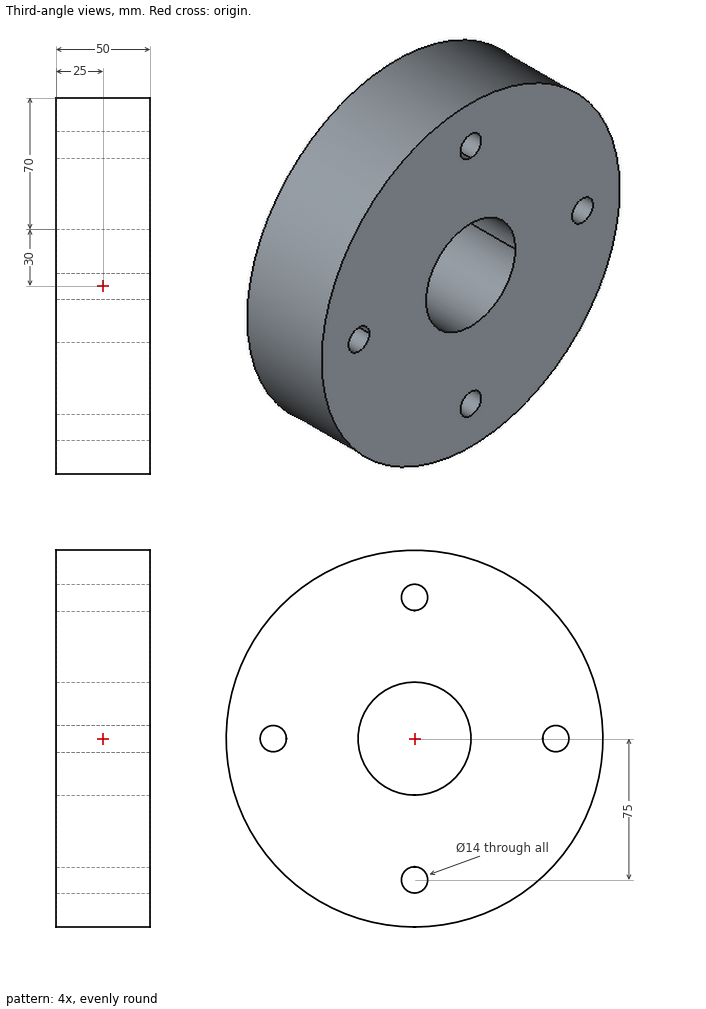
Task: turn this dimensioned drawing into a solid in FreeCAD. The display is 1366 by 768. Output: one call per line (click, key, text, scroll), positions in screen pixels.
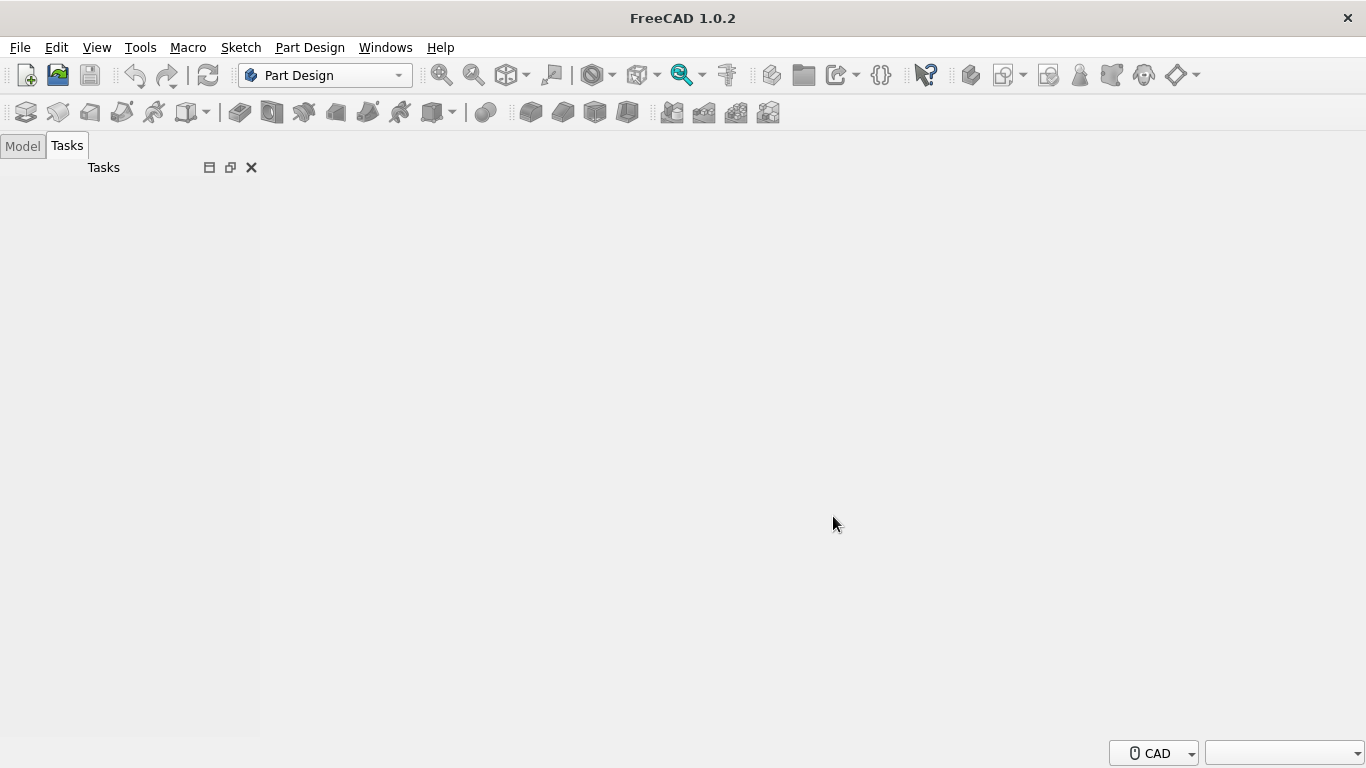
click(26, 76)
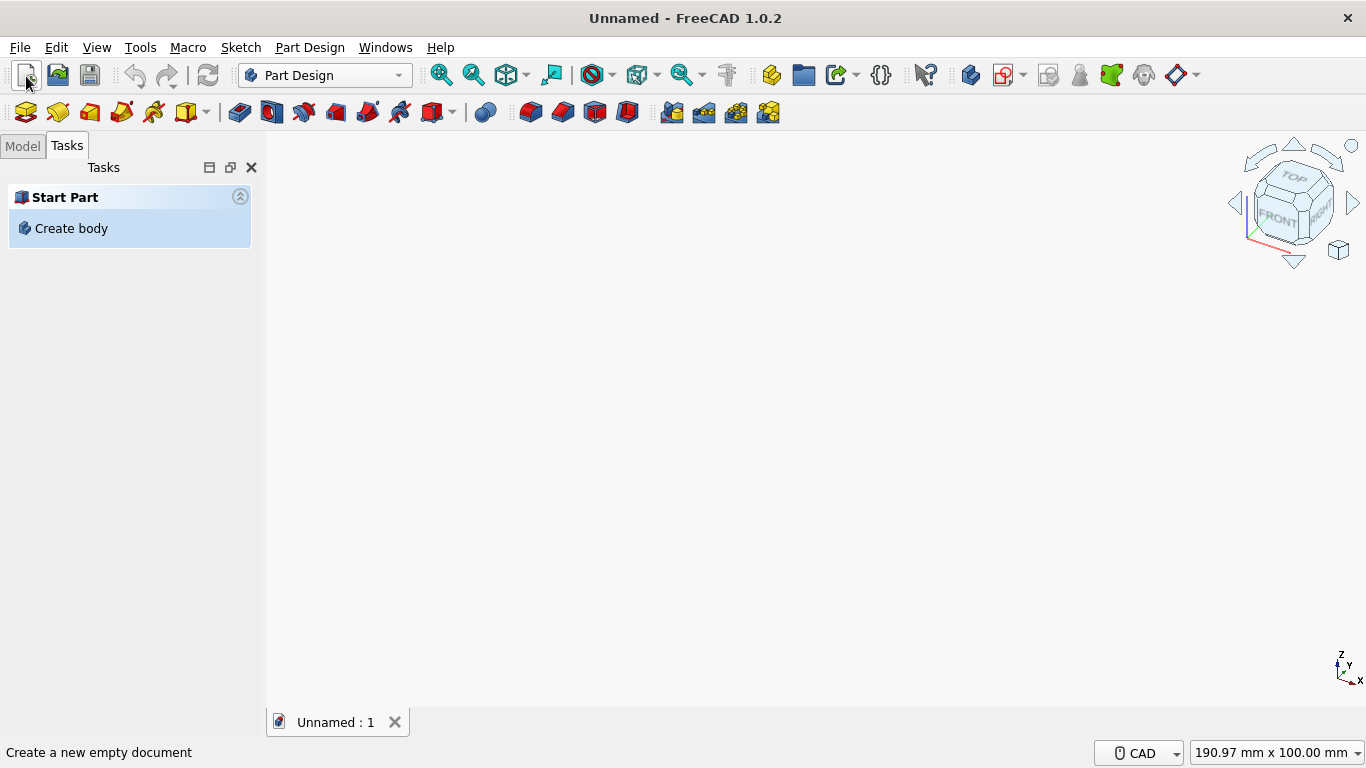
click(1004, 76)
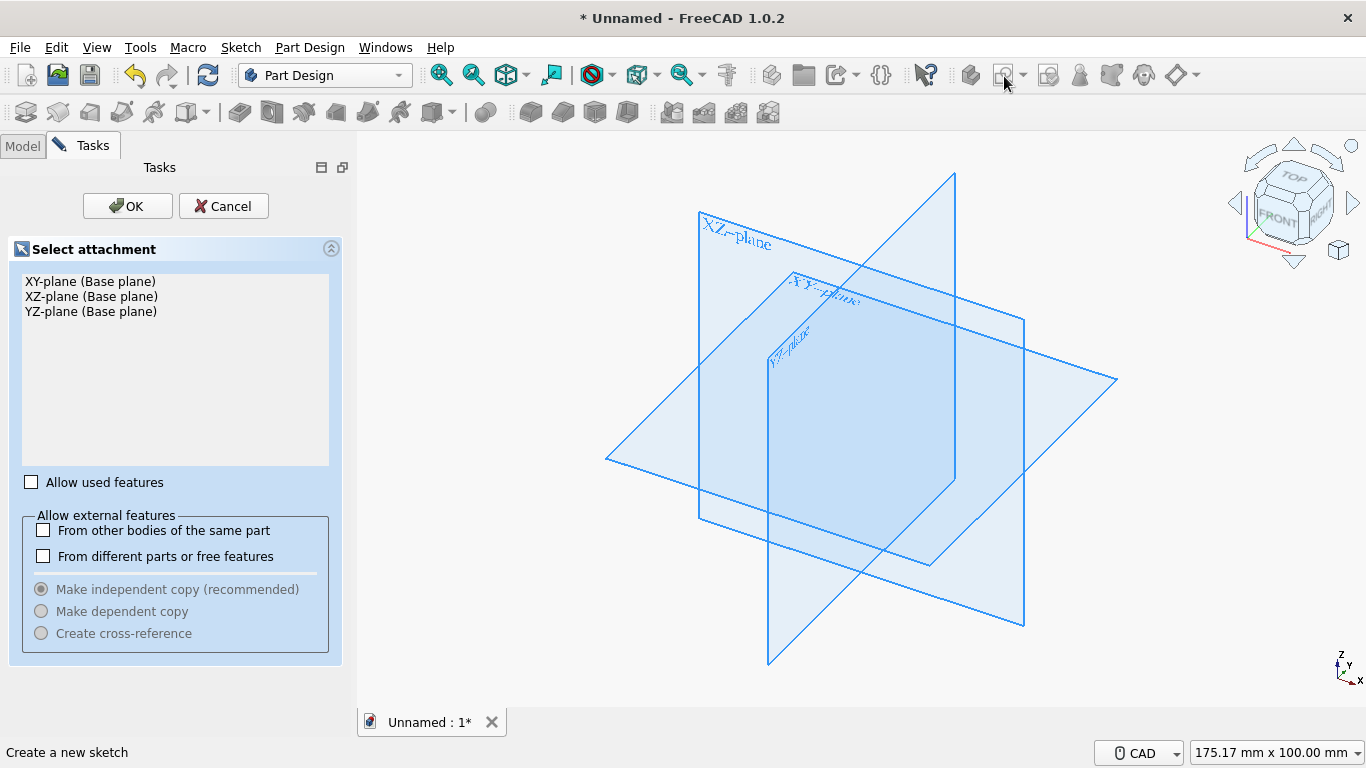
click(82, 282)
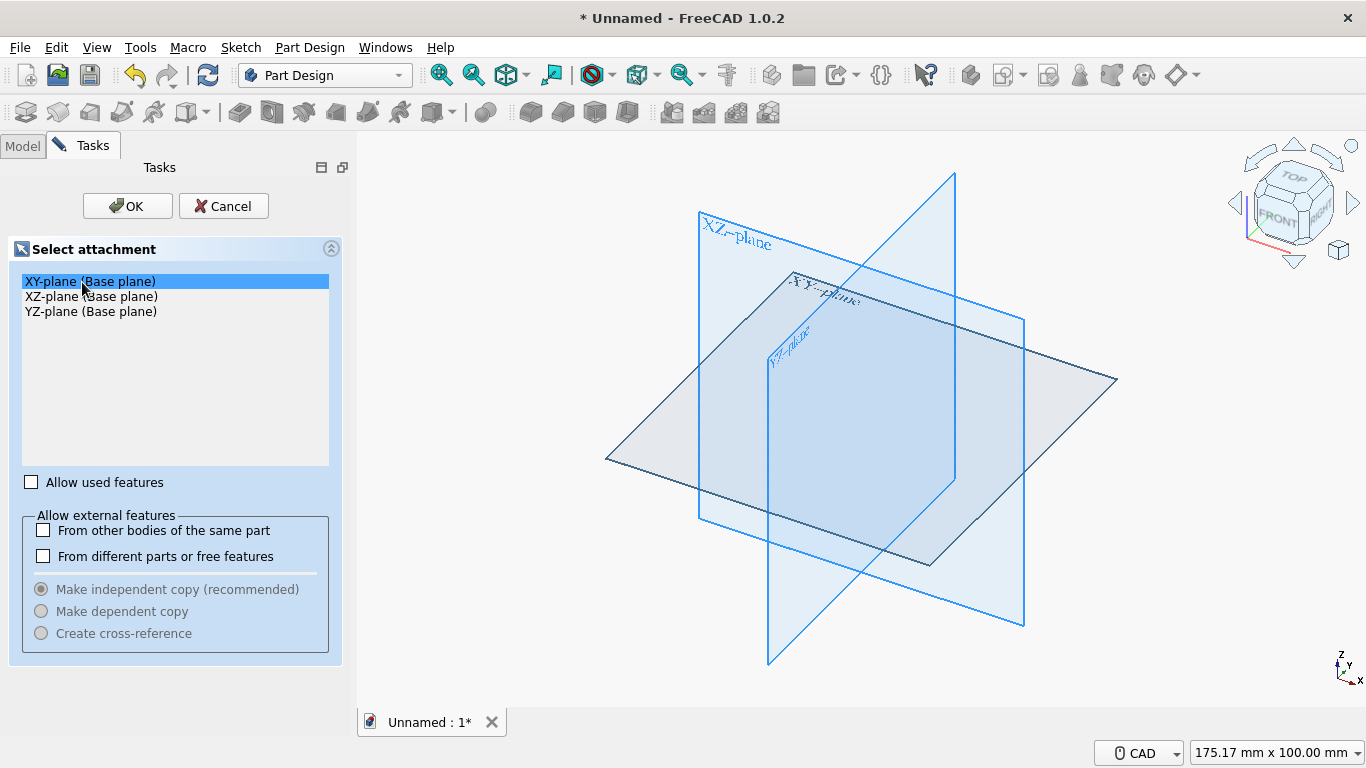
click(128, 206)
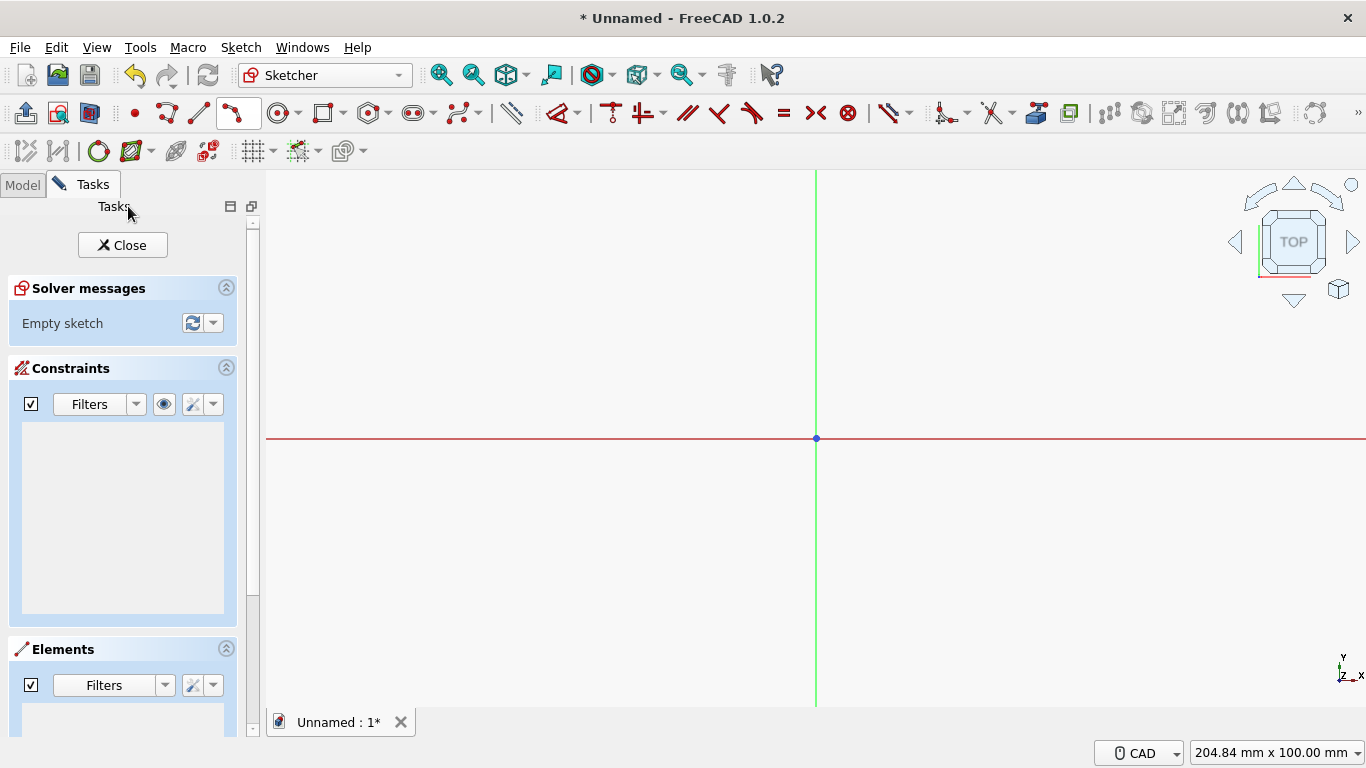
scroll(664, 679, down, 3)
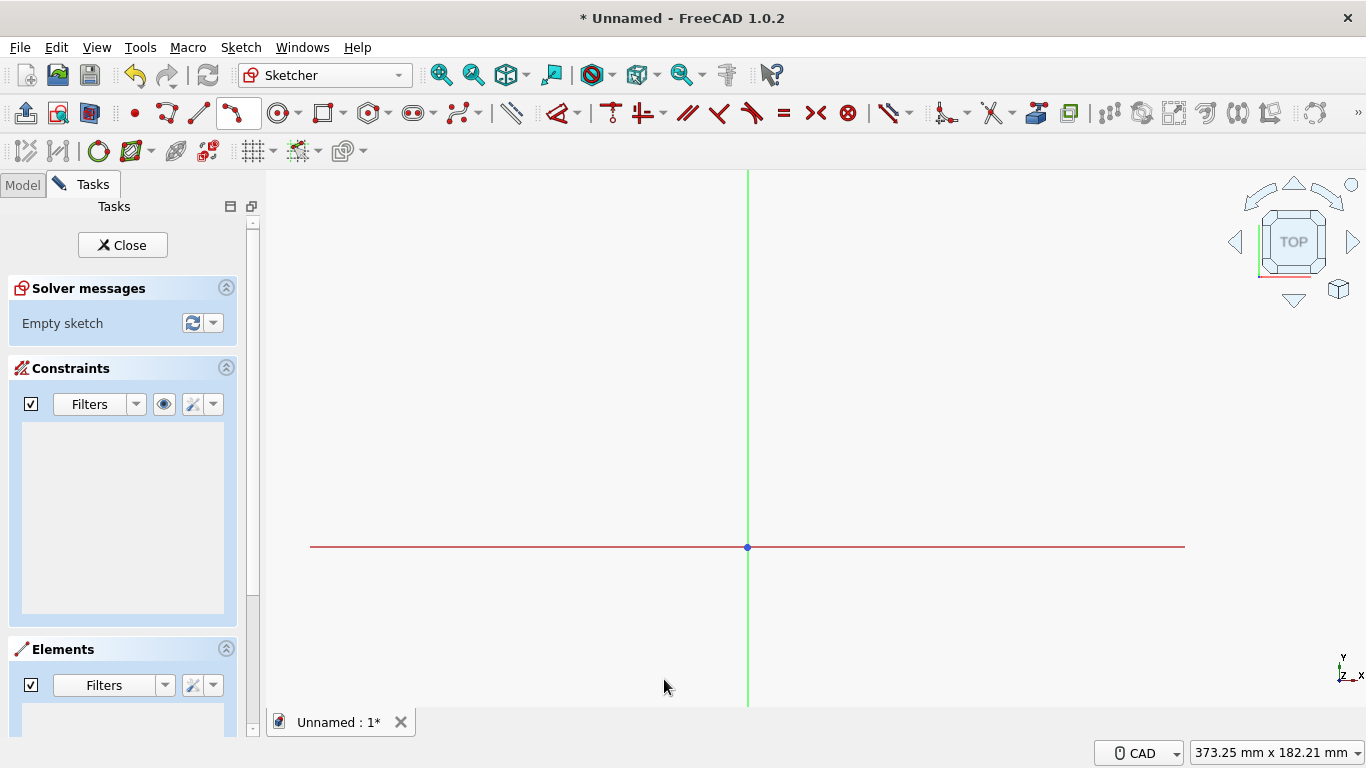
click(324, 114)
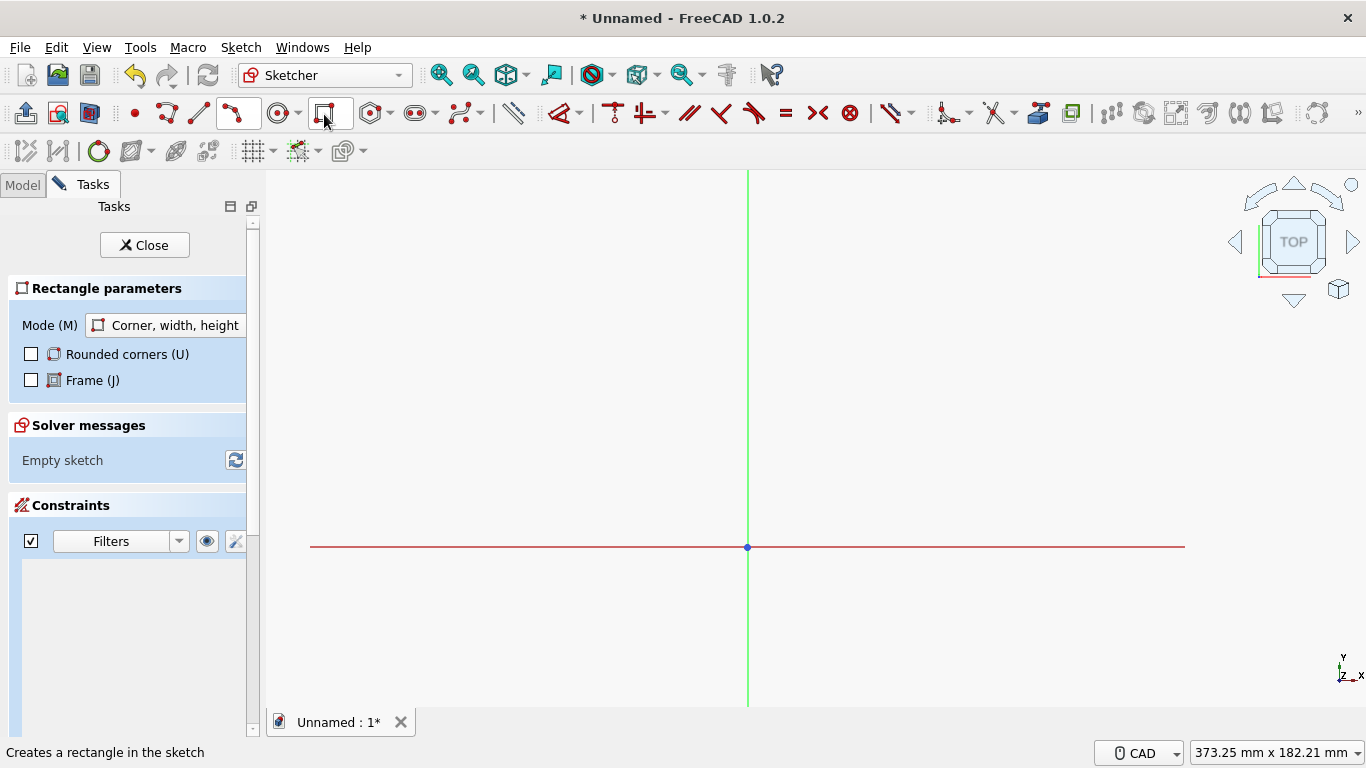
click(674, 253)
click(821, 459)
key(Escape)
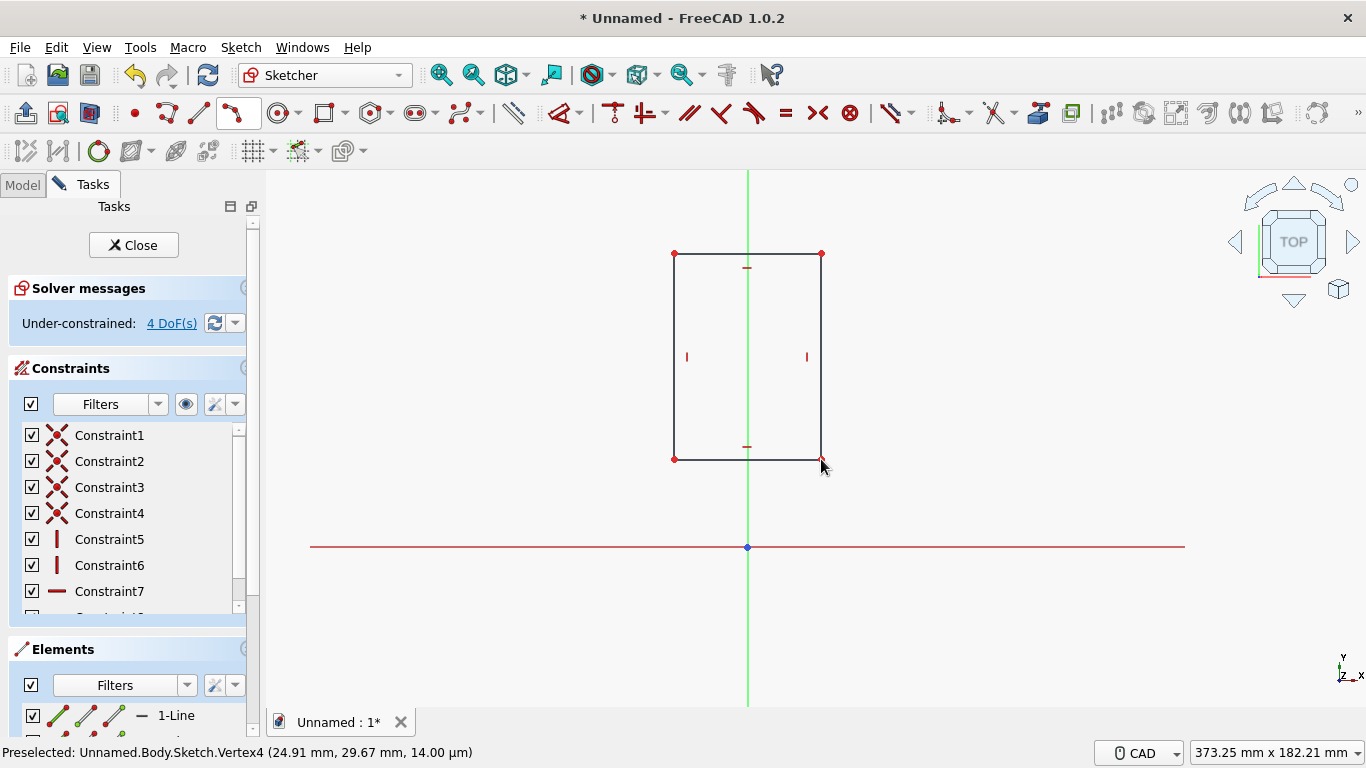
click(560, 114)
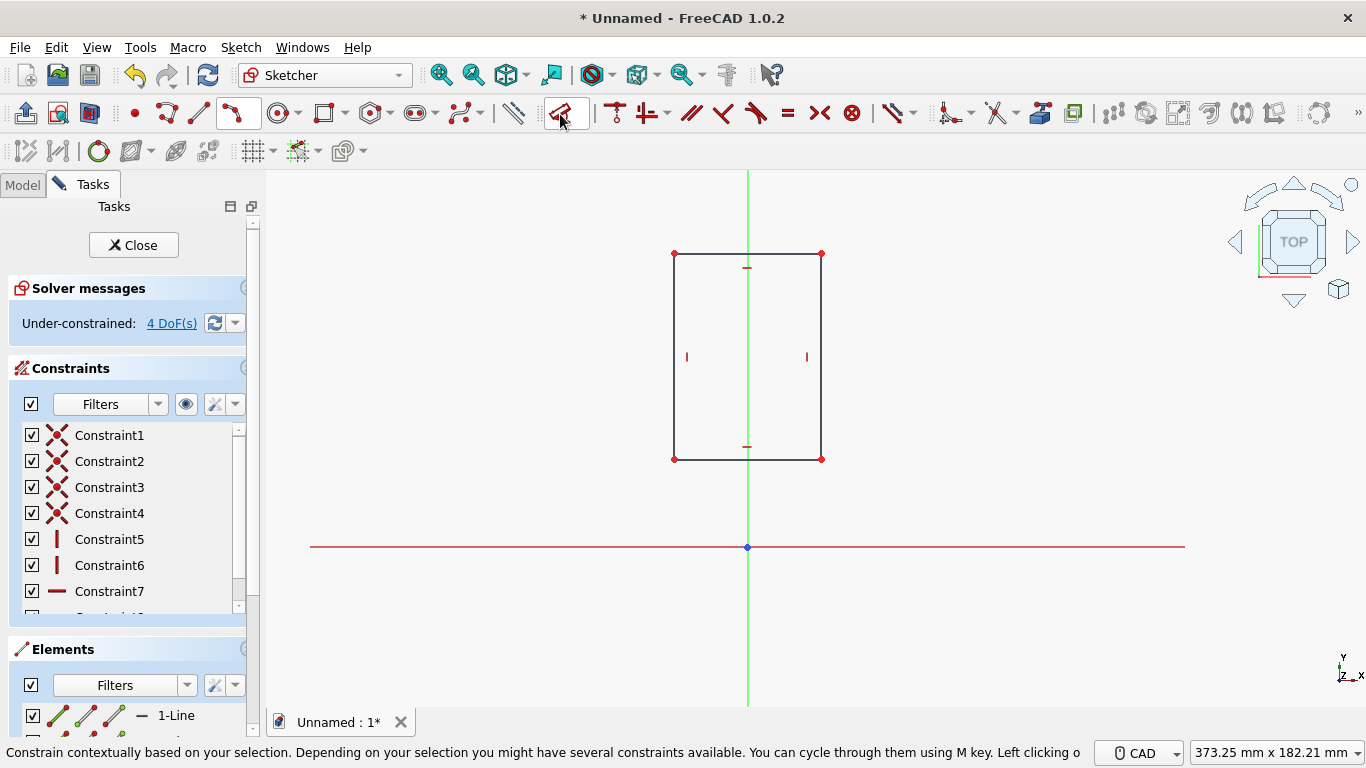
click(674, 316)
click(640, 357)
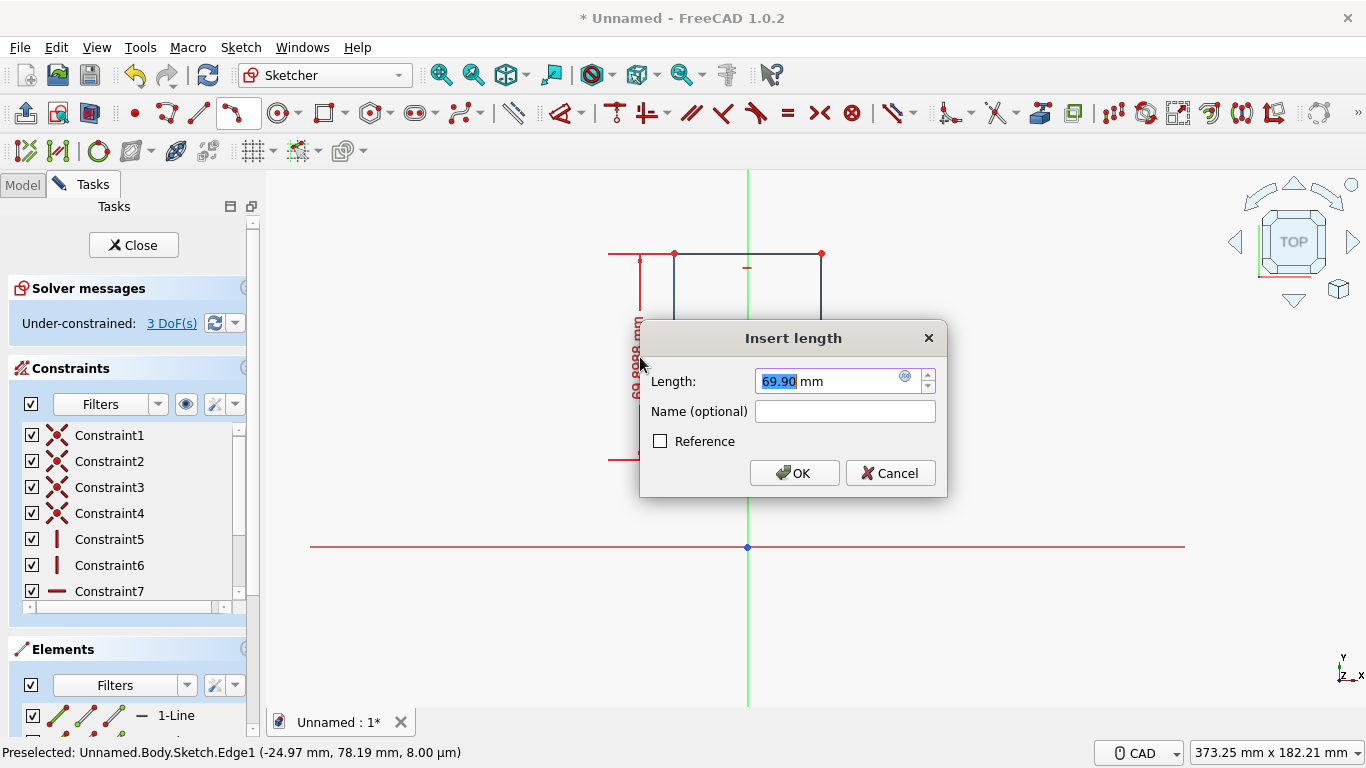
text(70)
key(Return)